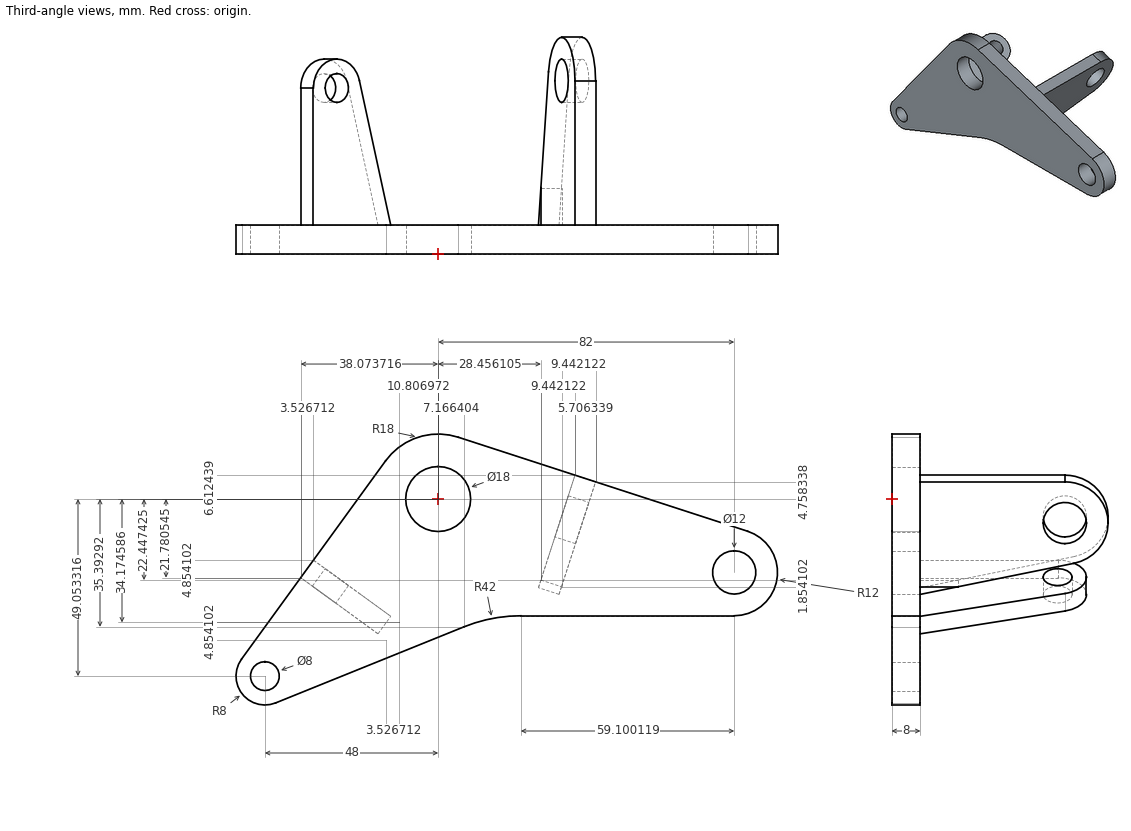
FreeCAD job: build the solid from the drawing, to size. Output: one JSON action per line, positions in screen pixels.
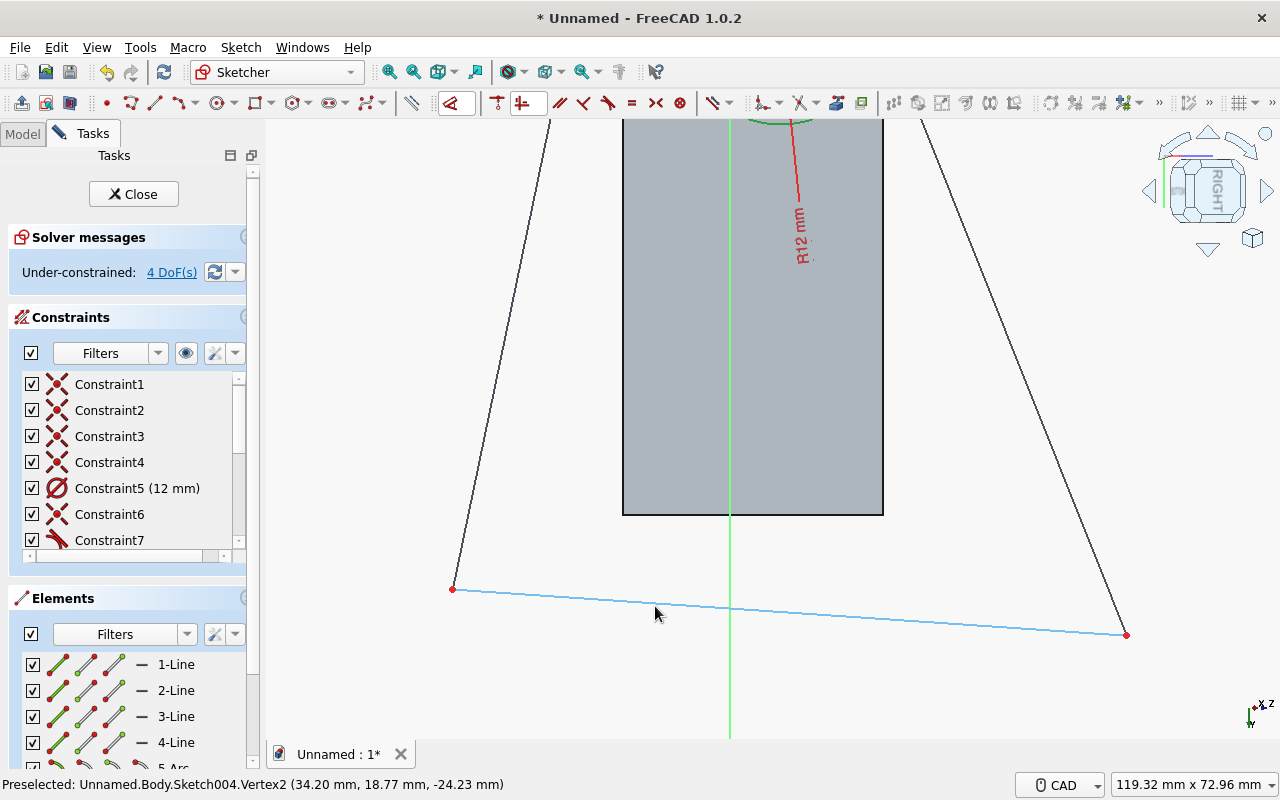
{"action": "left_click", "coordinate": [655, 603]}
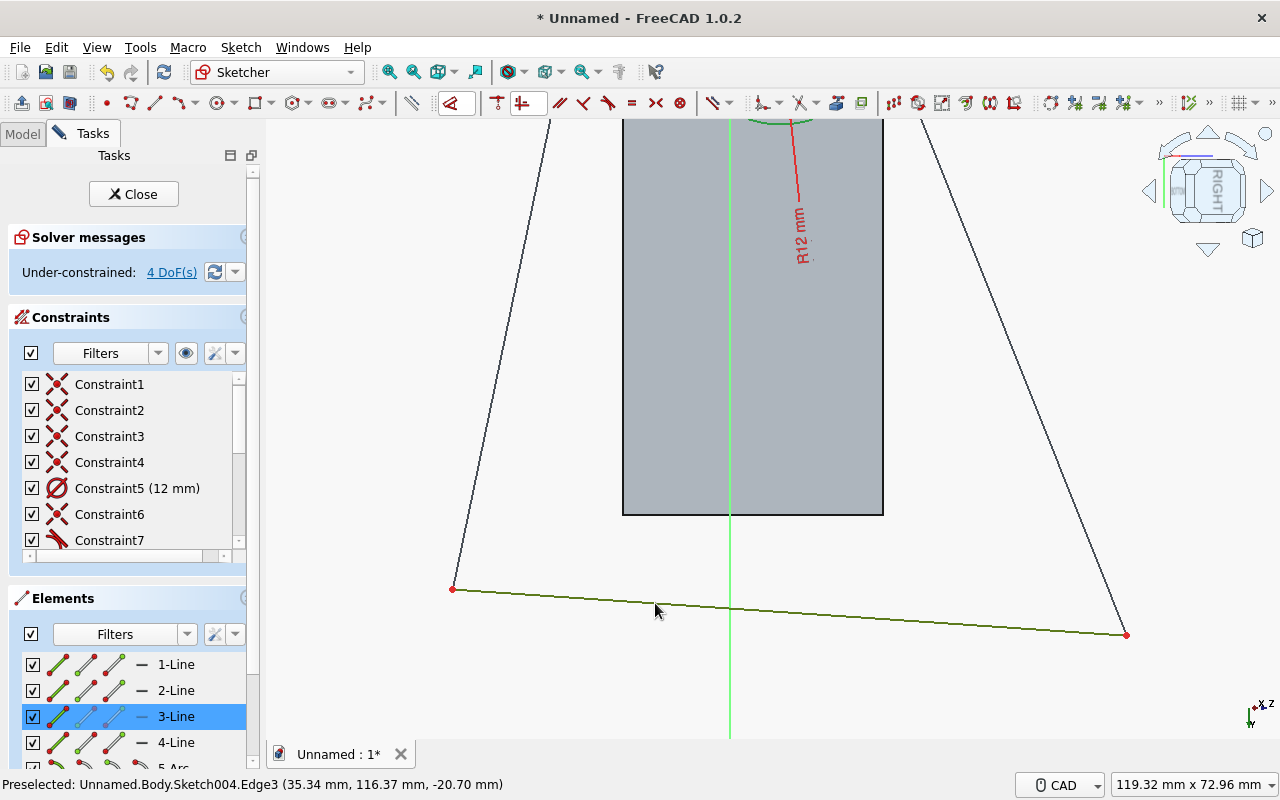
{"action": "left_click", "coordinate": [470, 104]}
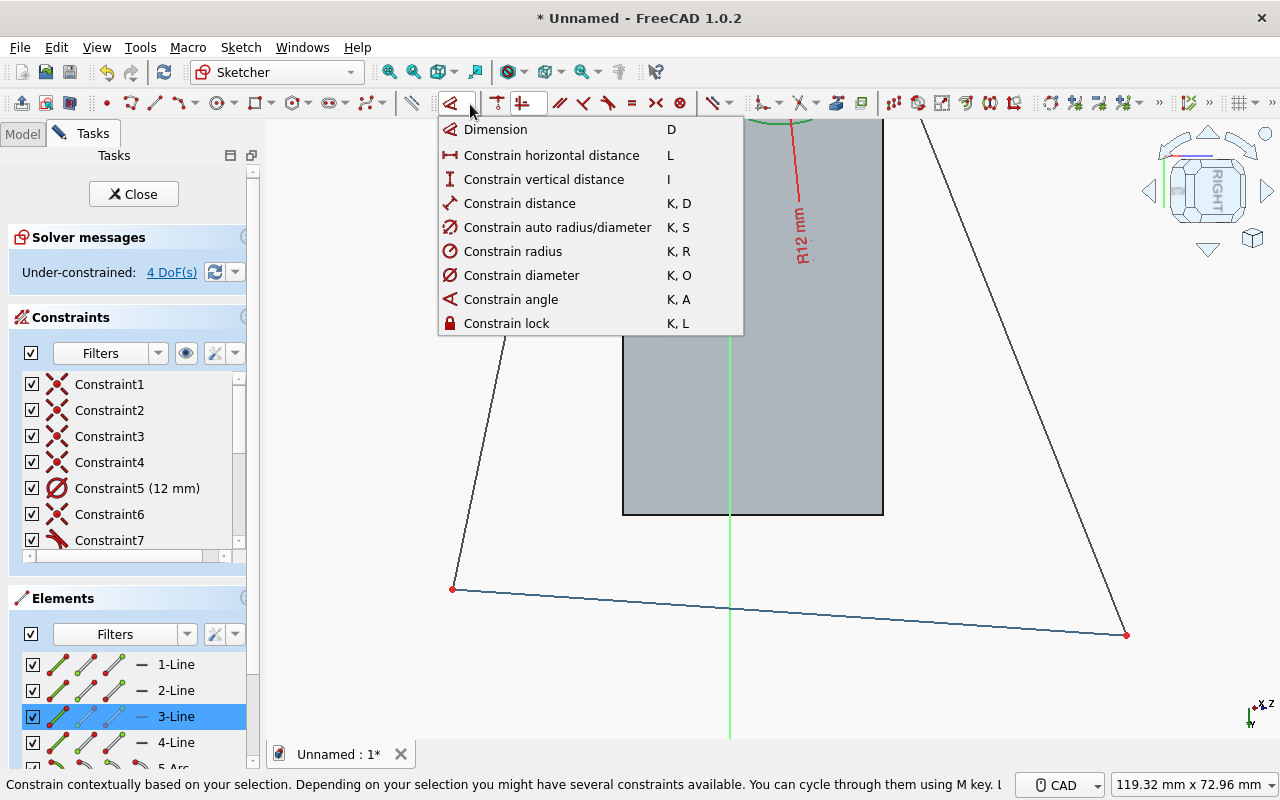
{"action": "left_click", "coordinate": [591, 179]}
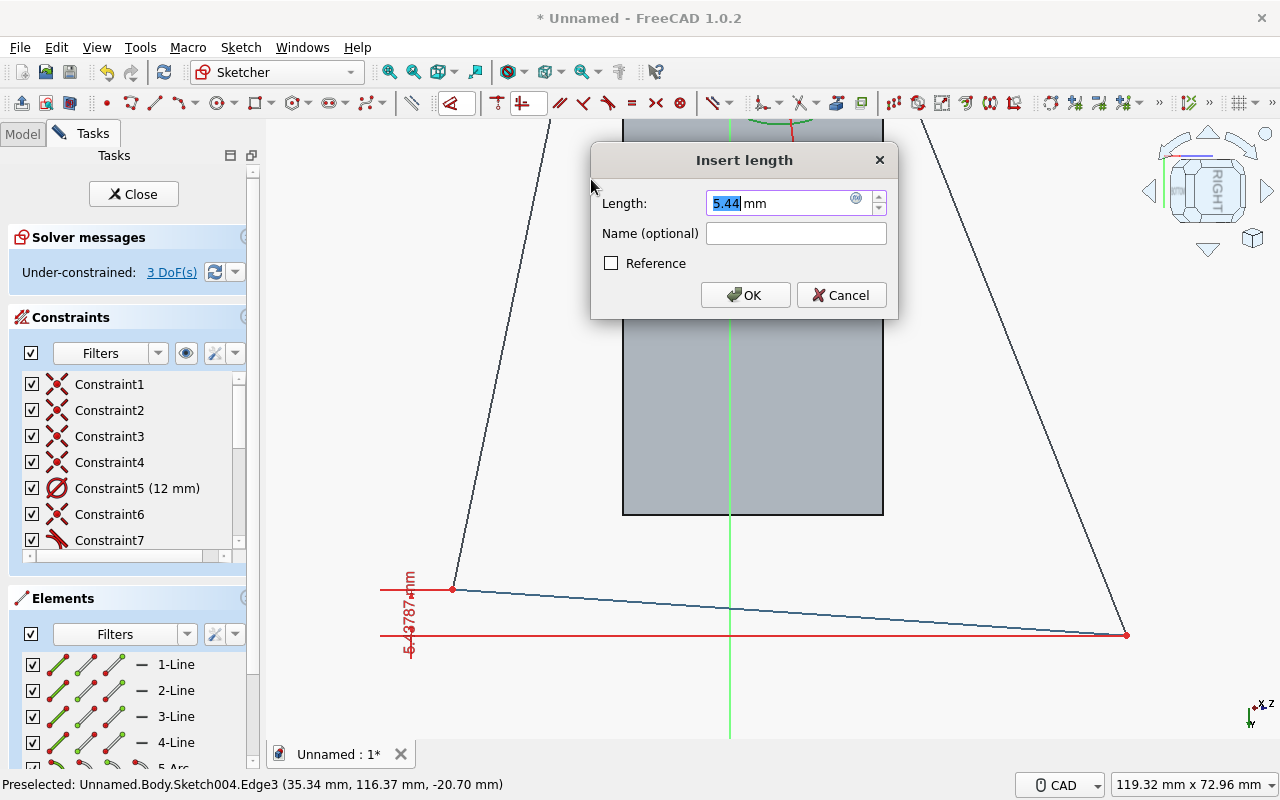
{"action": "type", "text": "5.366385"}
{"action": "key", "text": "Return"}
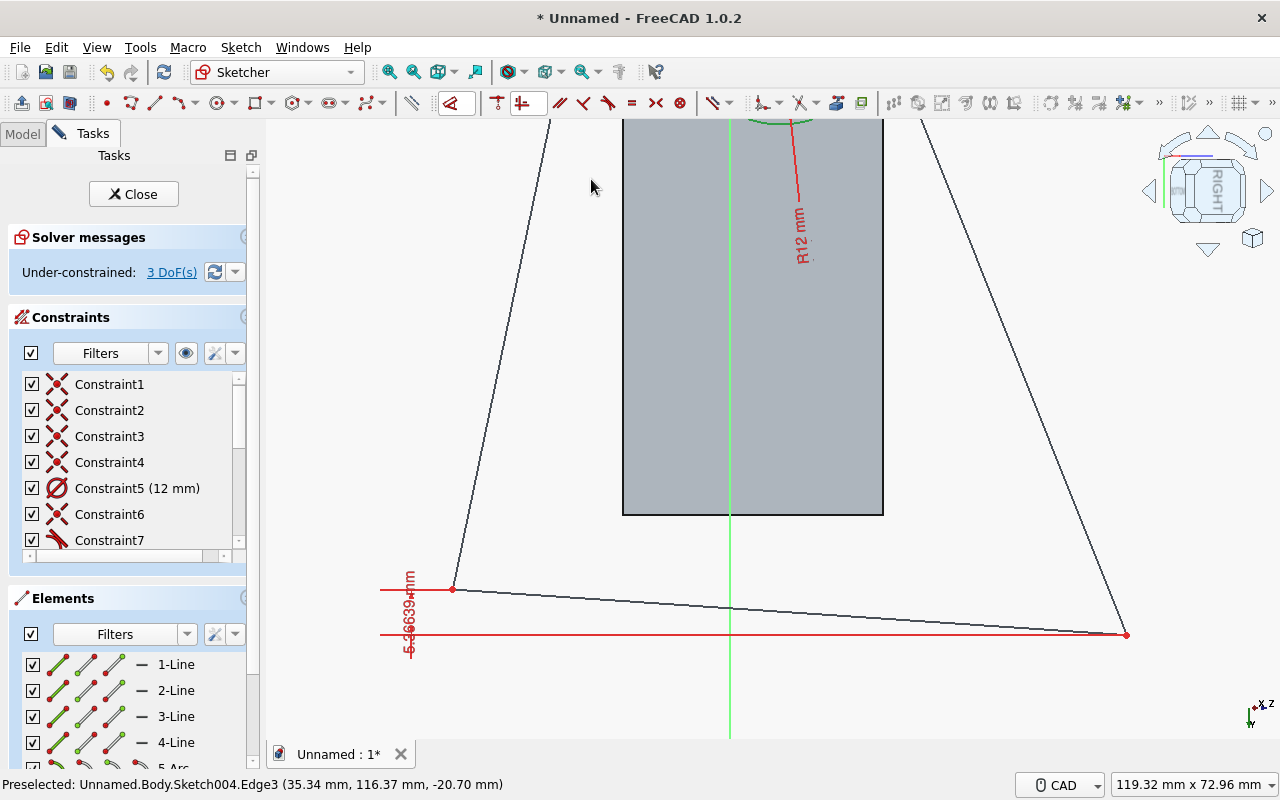
{"action": "left_click", "coordinate": [453, 590]}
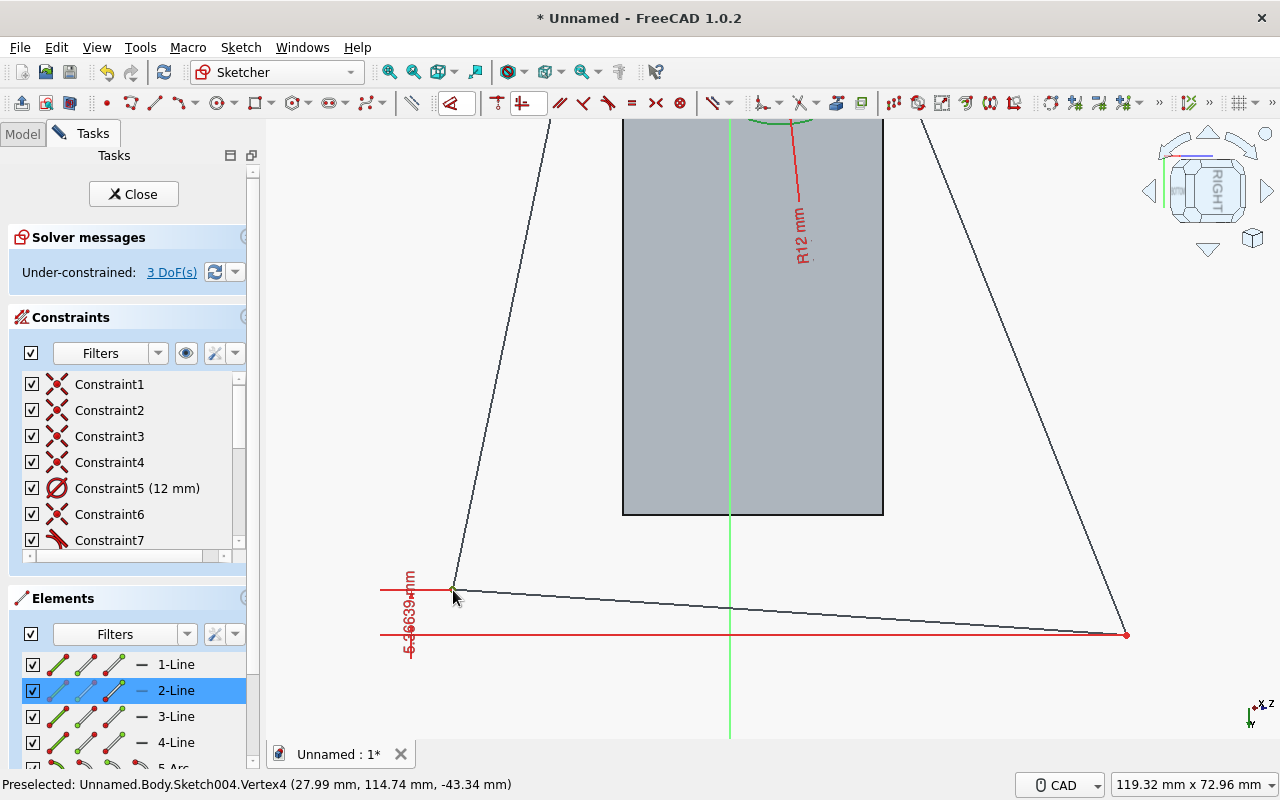
{"action": "left_click", "coordinate": [470, 104]}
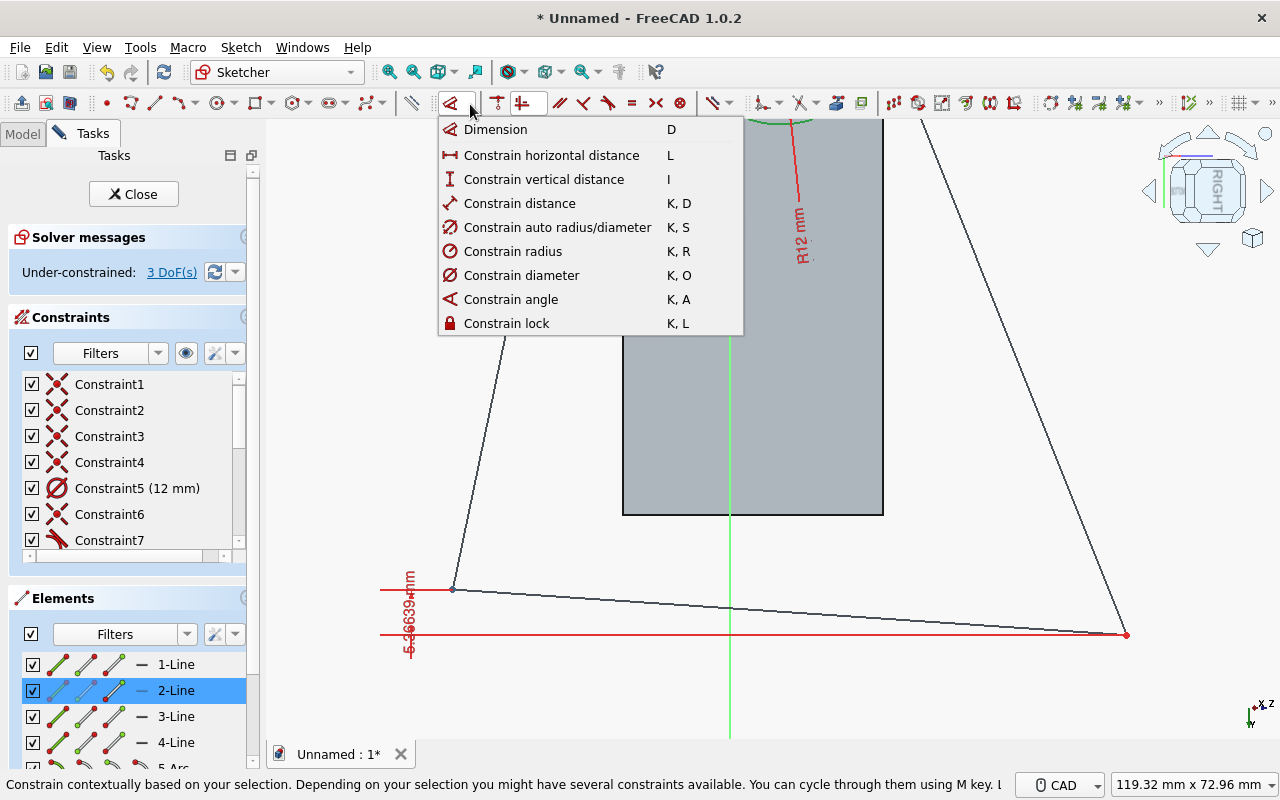
{"action": "left_click", "coordinate": [591, 155]}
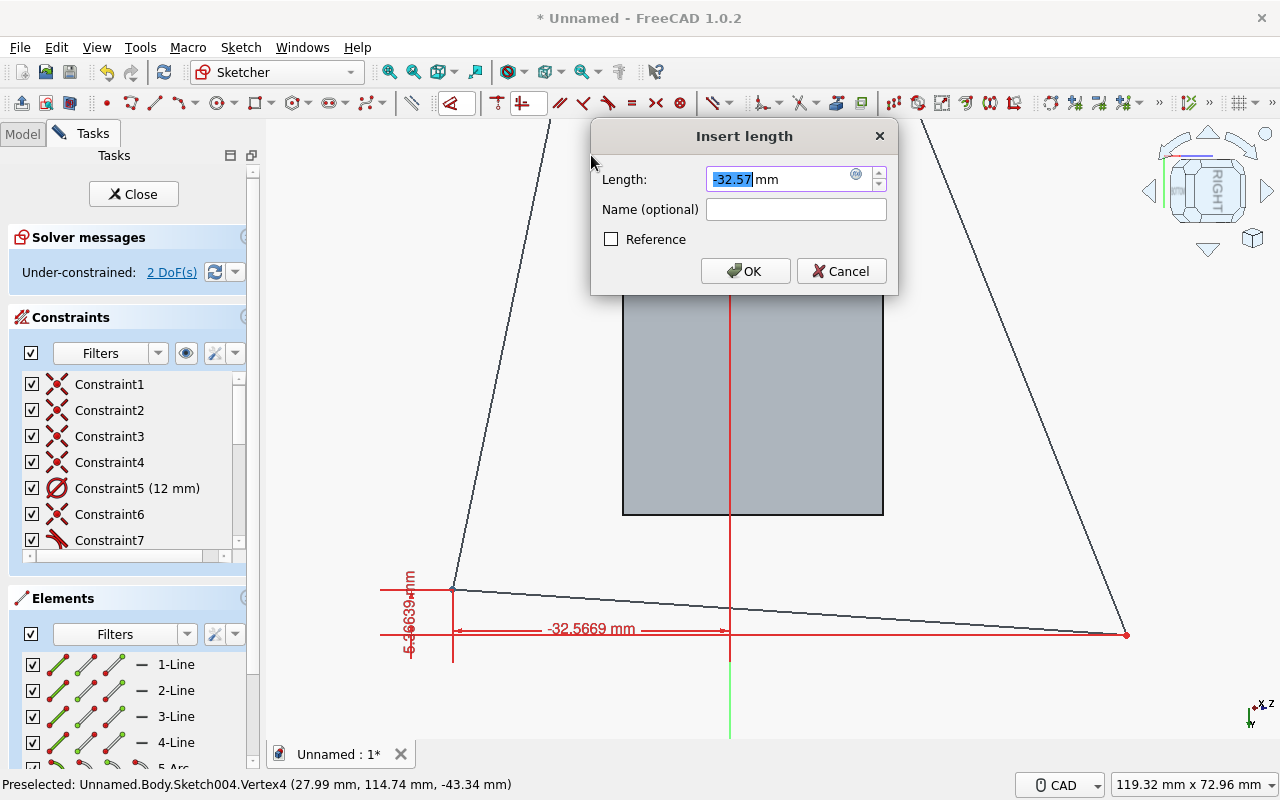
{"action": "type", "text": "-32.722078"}
{"action": "key", "text": "Return"}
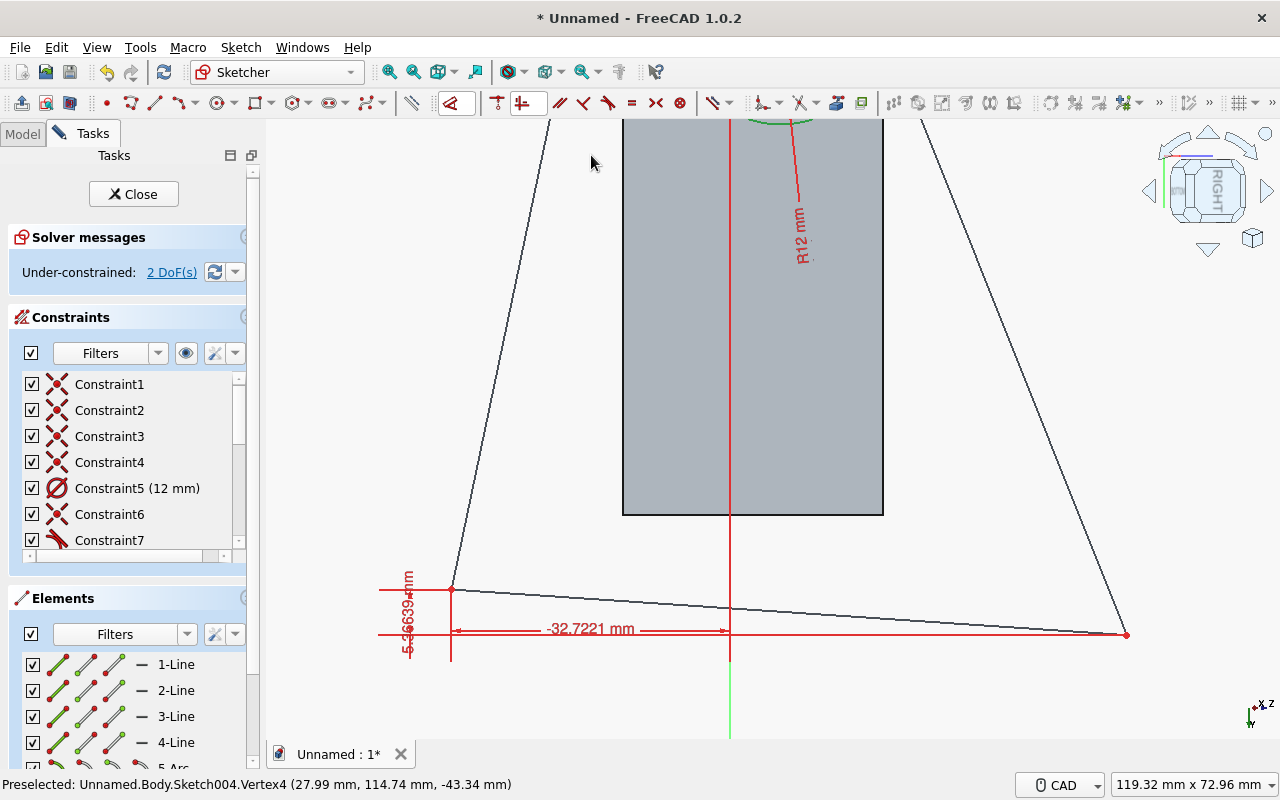
{"action": "left_click", "coordinate": [451, 590]}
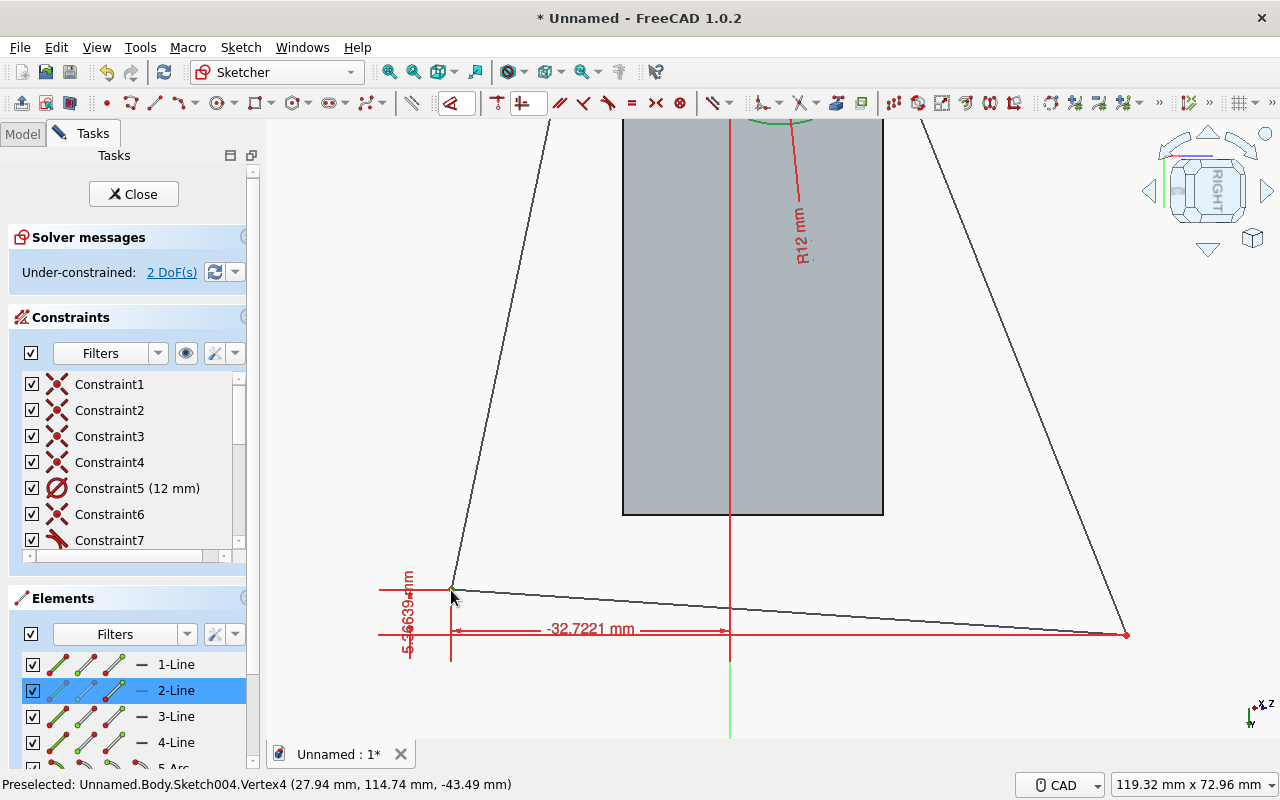
{"action": "left_click", "coordinate": [470, 104]}